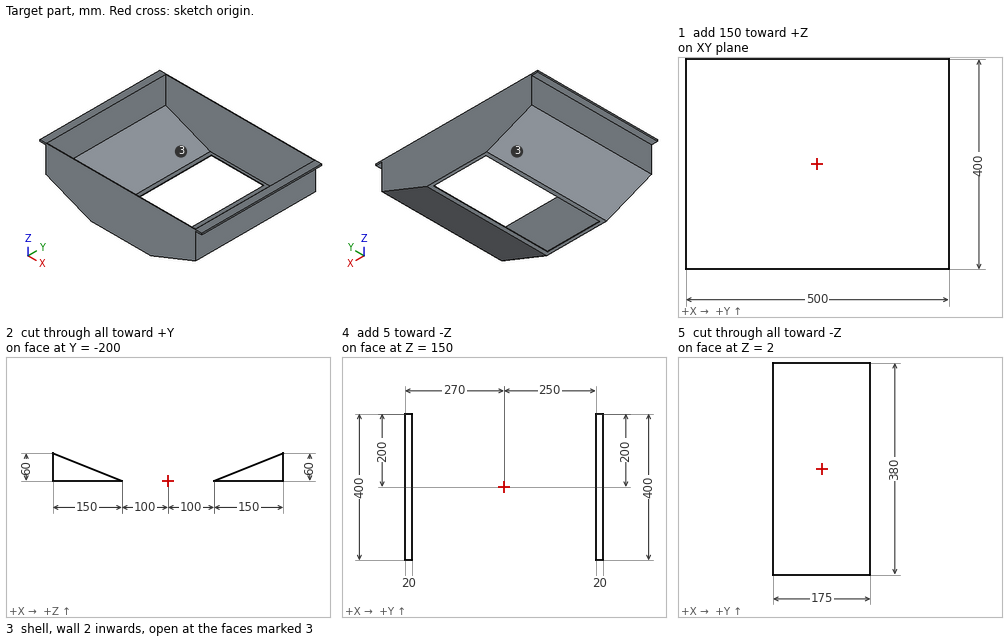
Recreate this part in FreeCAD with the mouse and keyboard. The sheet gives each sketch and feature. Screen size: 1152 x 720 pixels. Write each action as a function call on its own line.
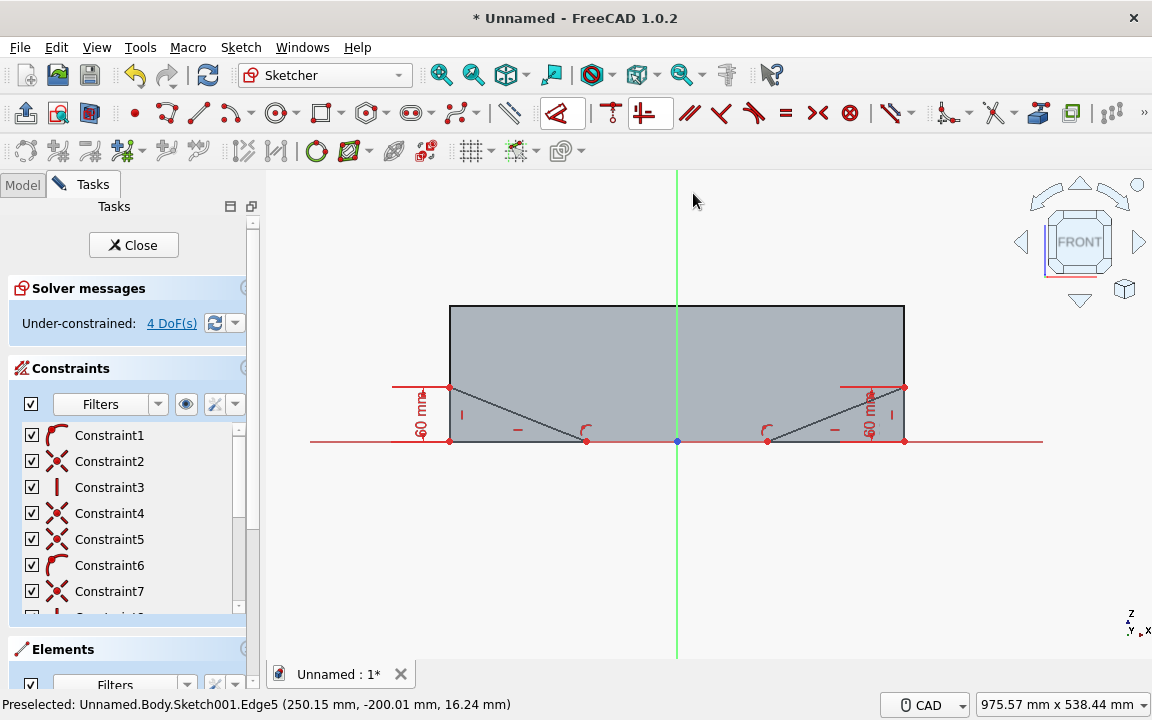
click(491, 442)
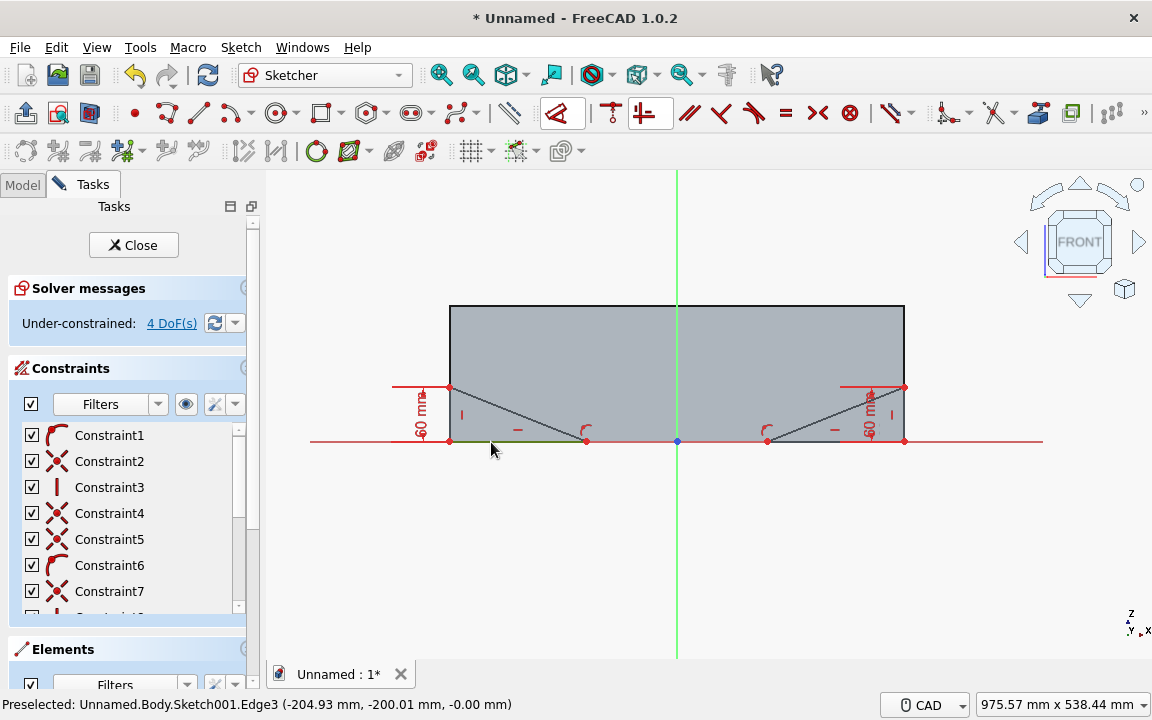
key(l)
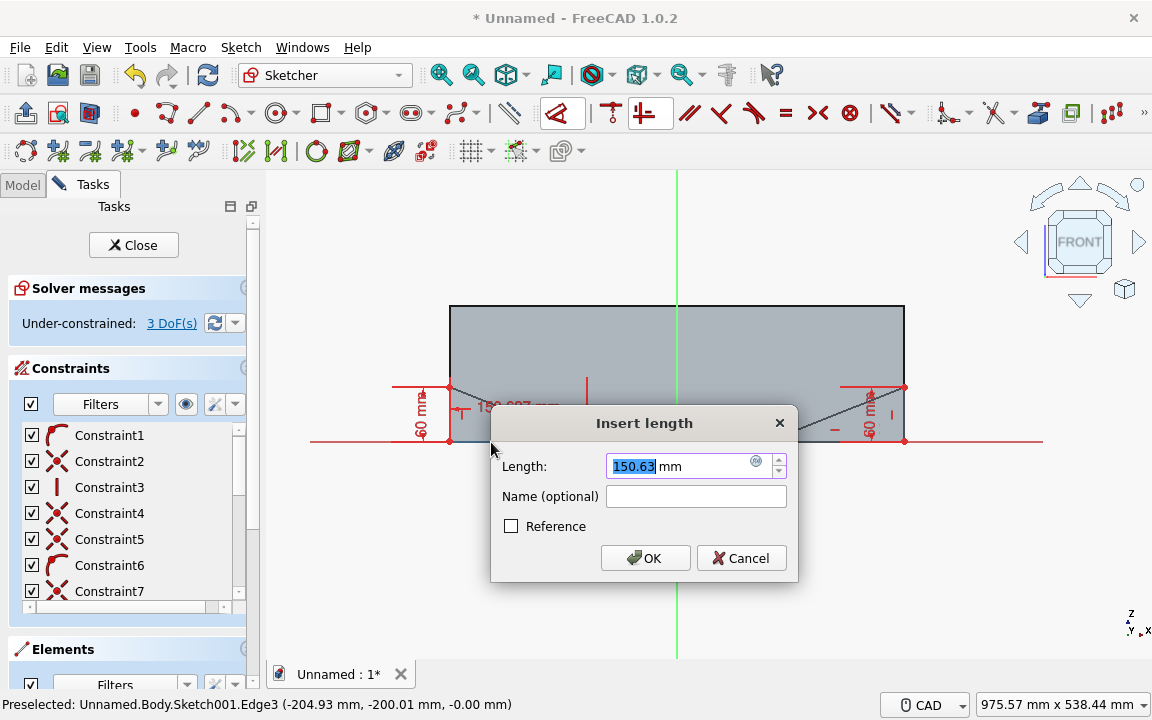
text(150)
key(Return)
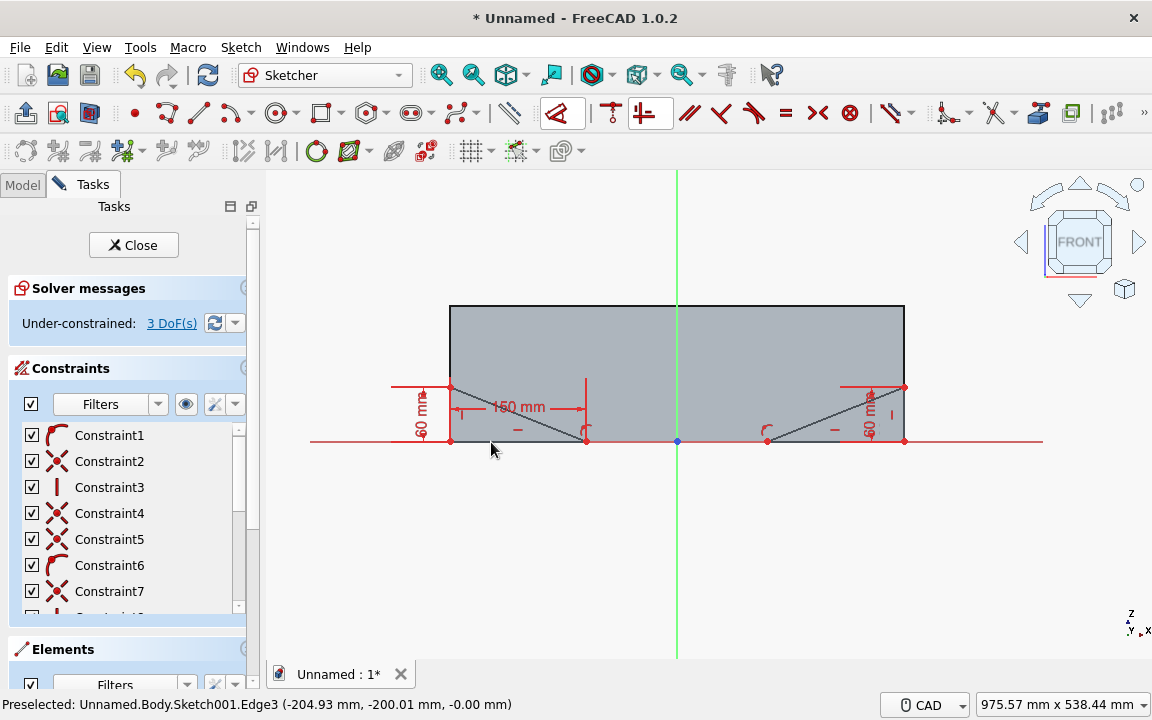
click(809, 442)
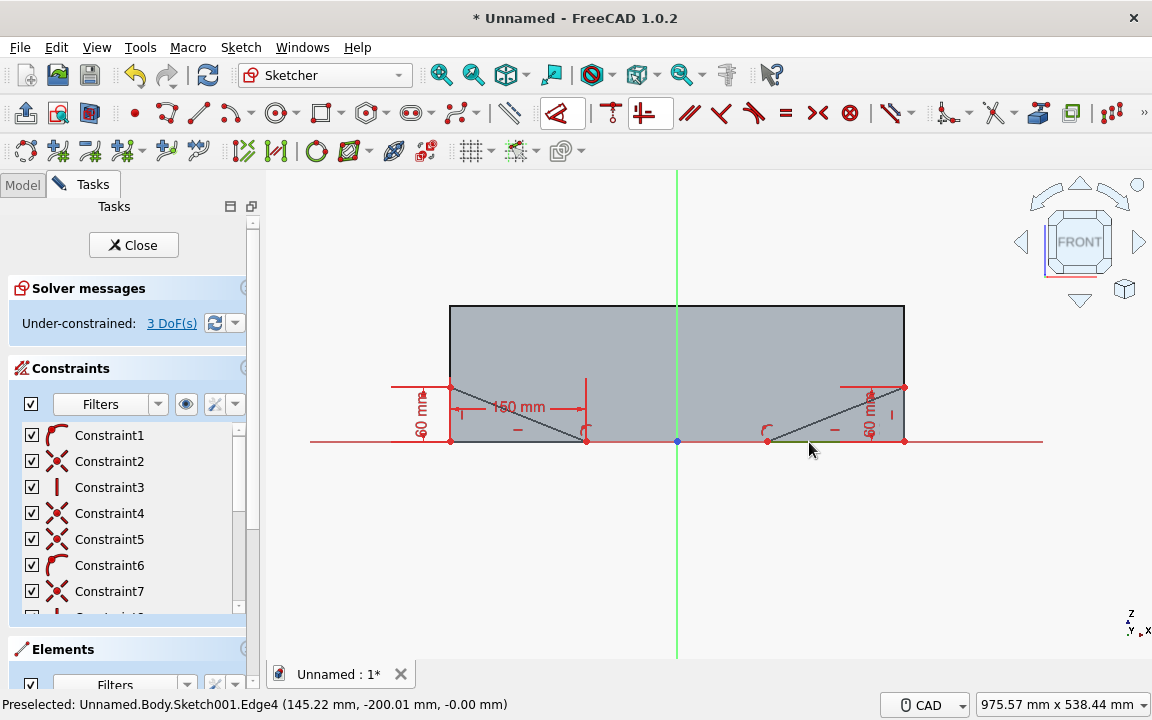
key(l)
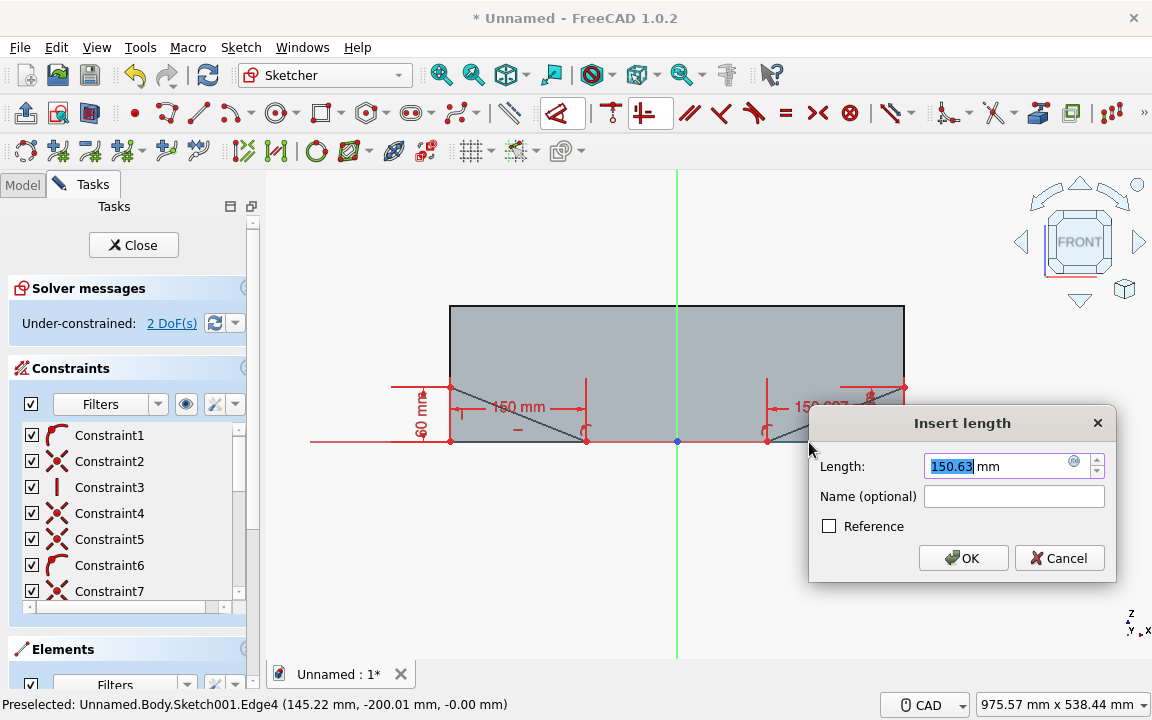
text(150)
key(Return)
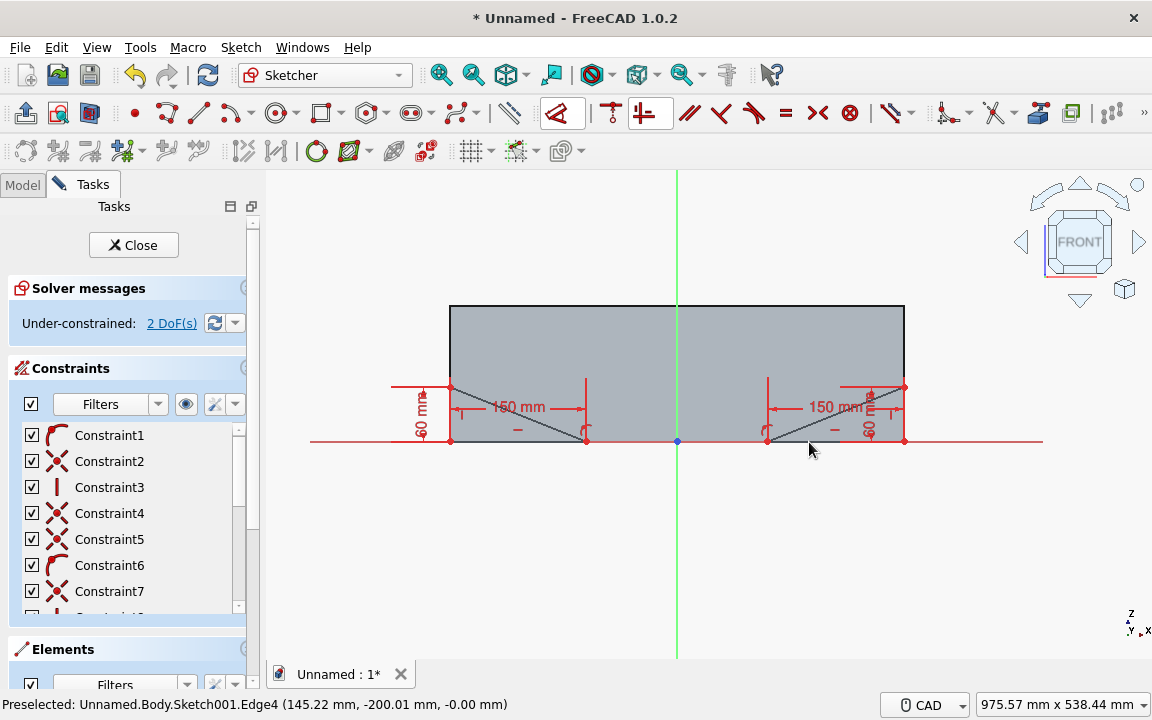
click(586, 442)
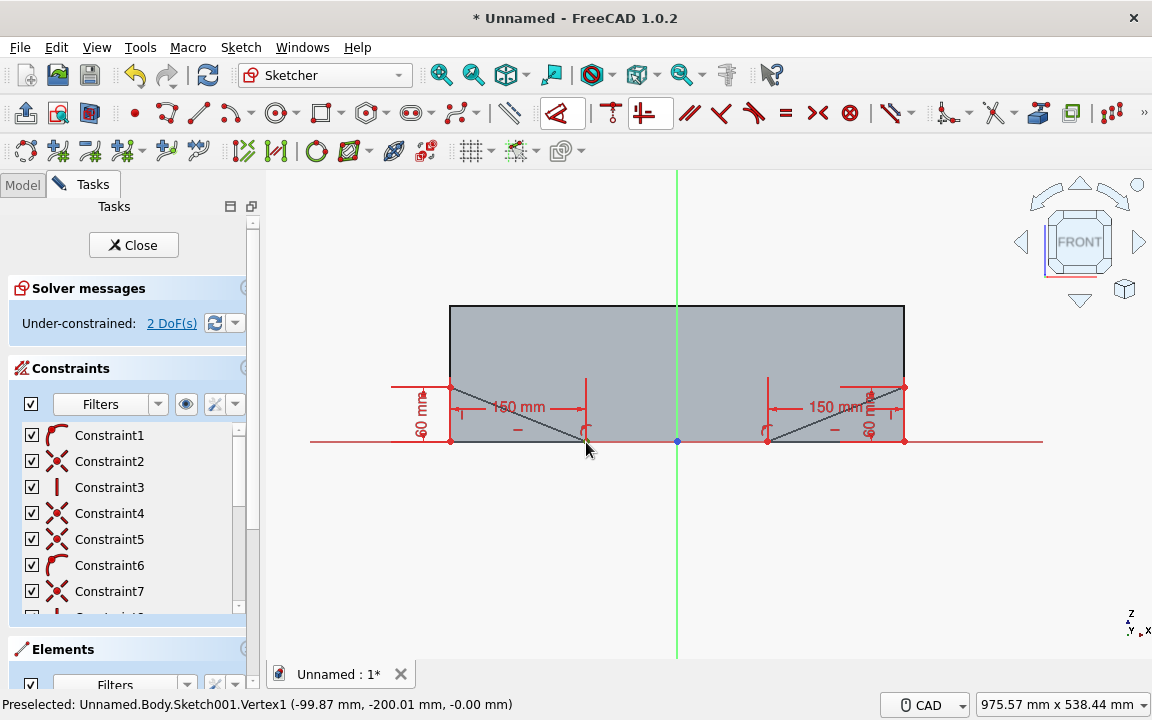
click(580, 114)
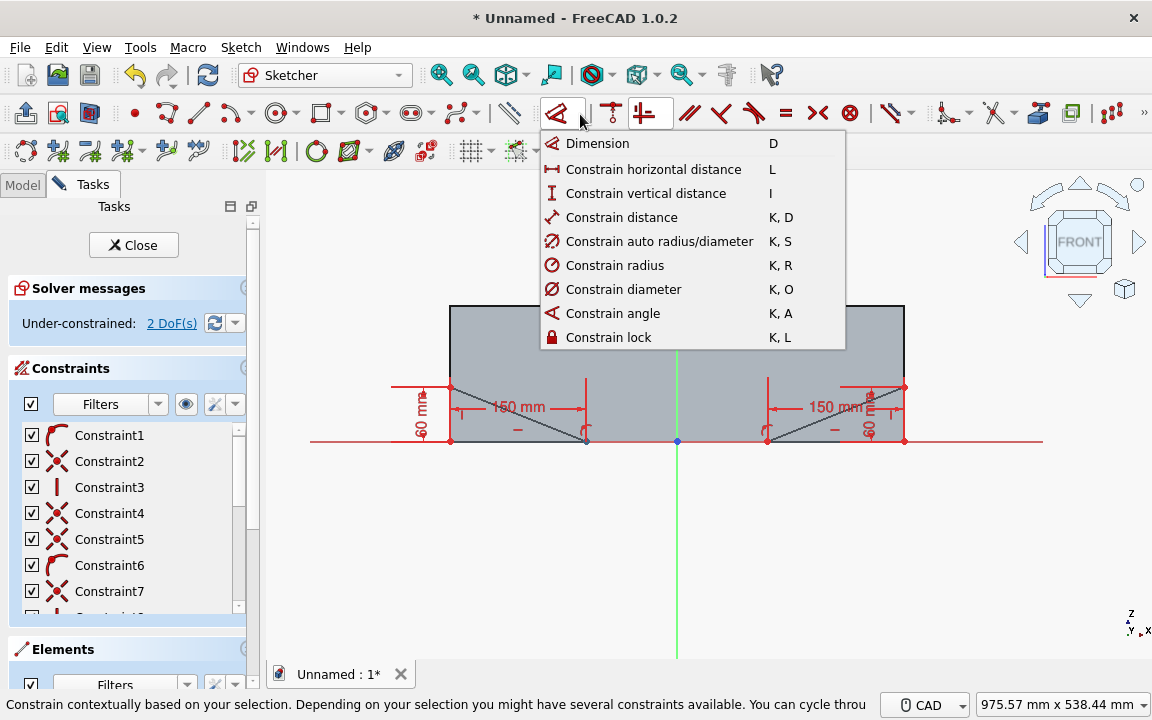
click(693, 169)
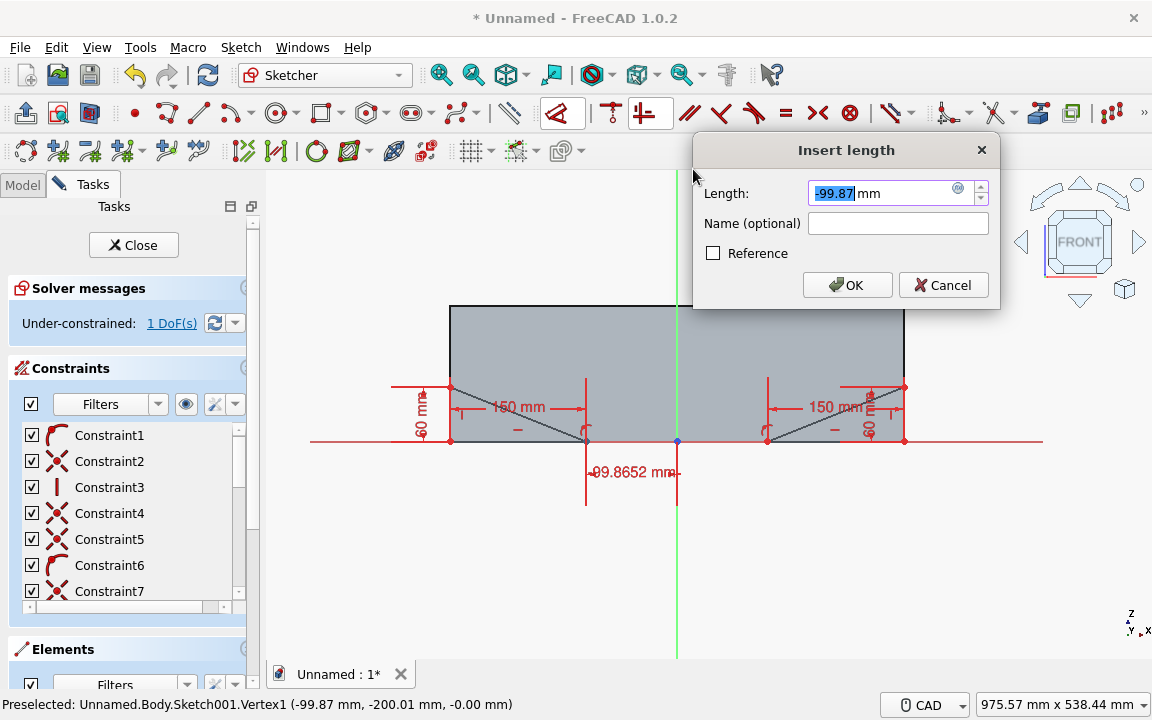
text(-100)
key(Return)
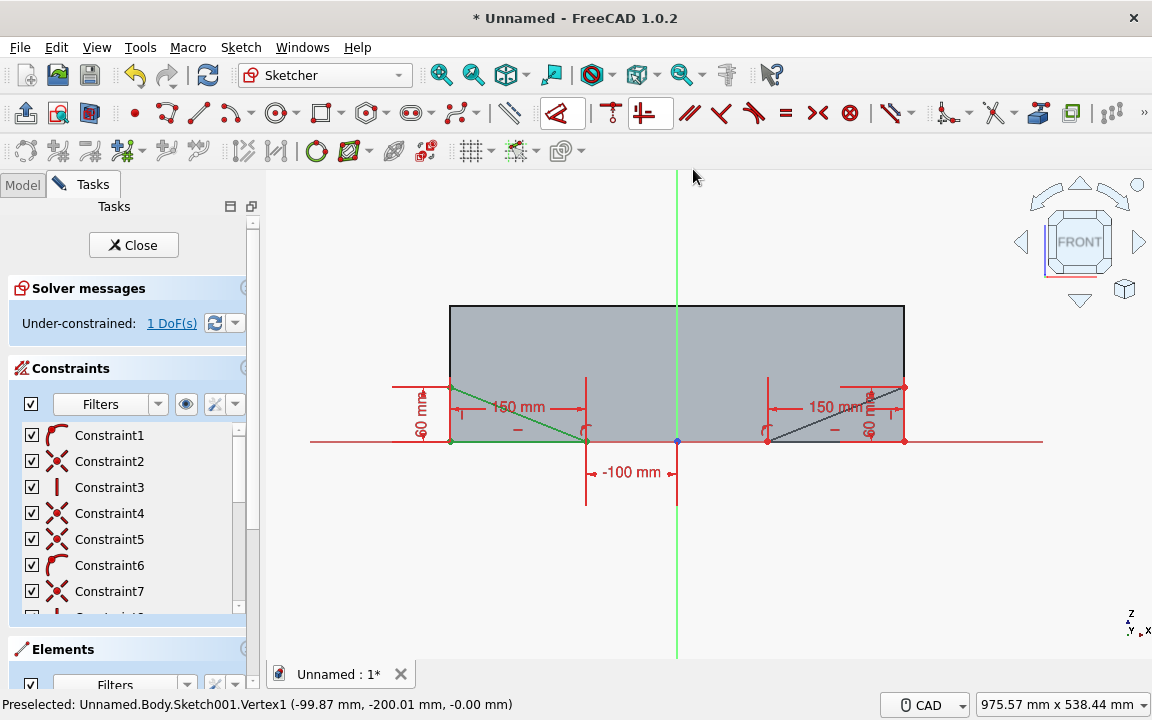
click(768, 442)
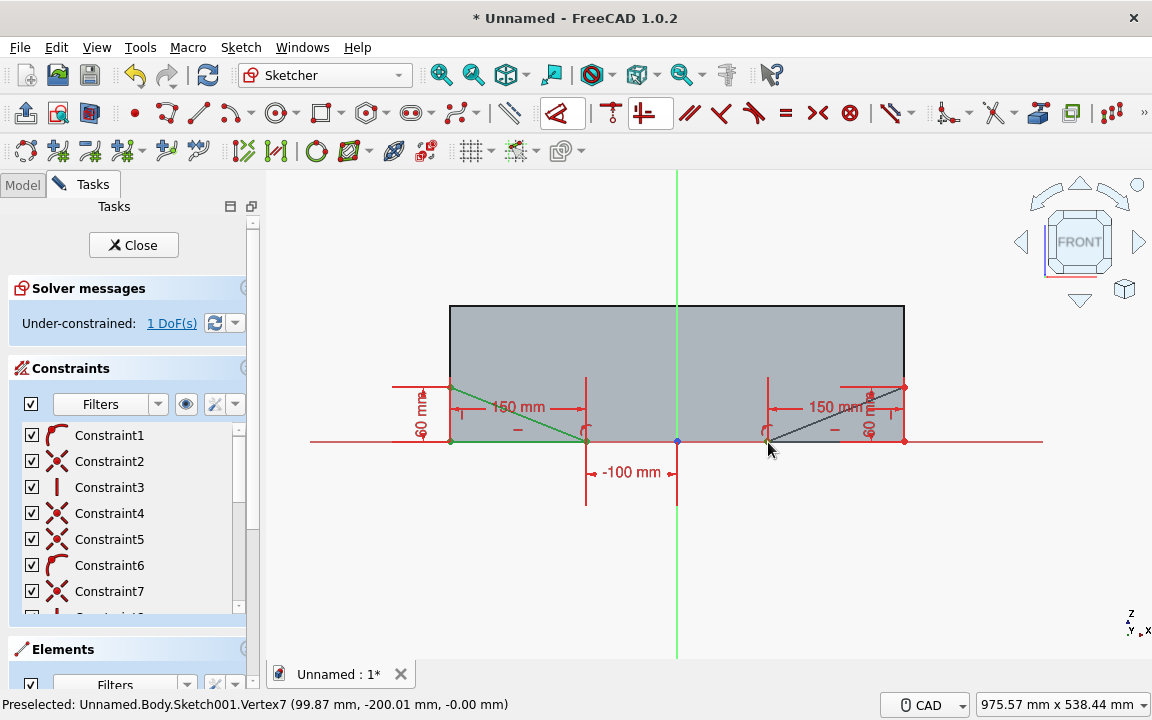
click(580, 114)